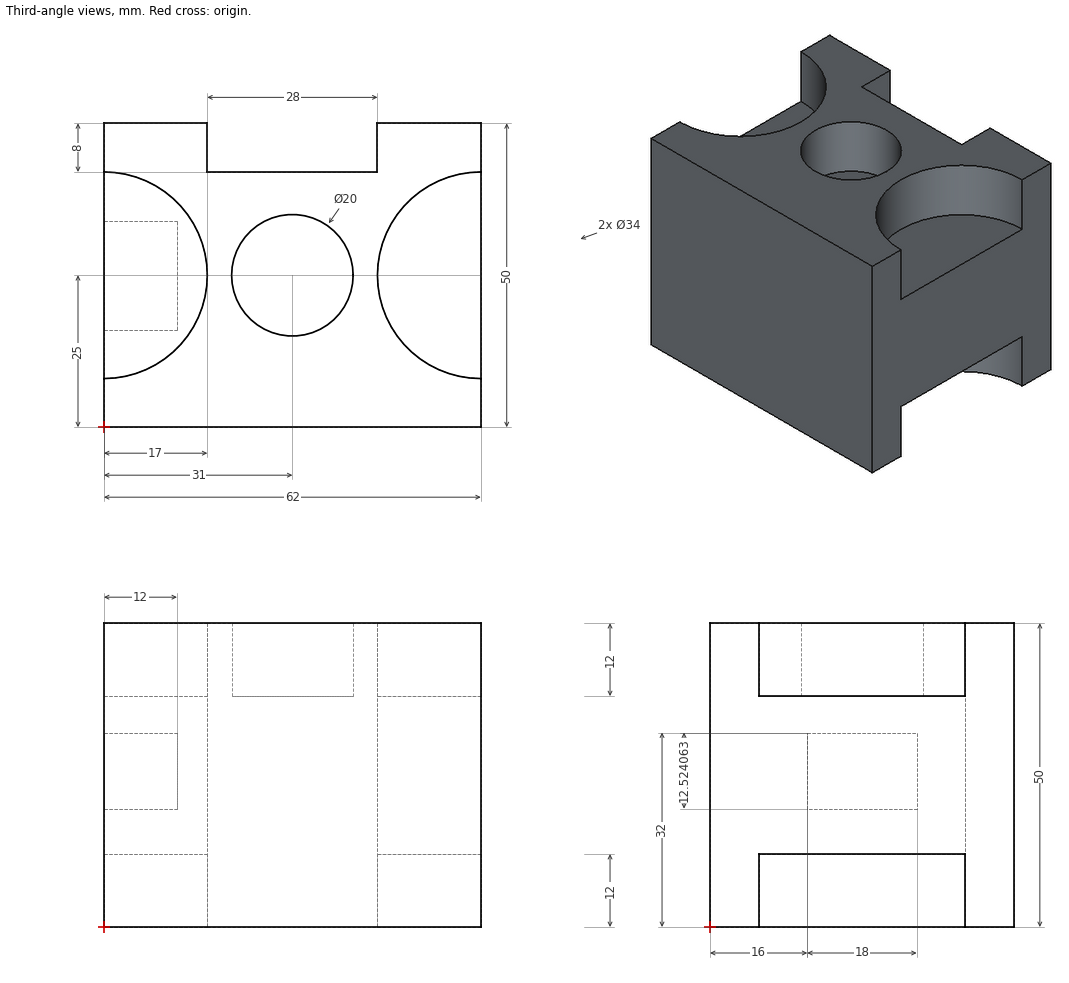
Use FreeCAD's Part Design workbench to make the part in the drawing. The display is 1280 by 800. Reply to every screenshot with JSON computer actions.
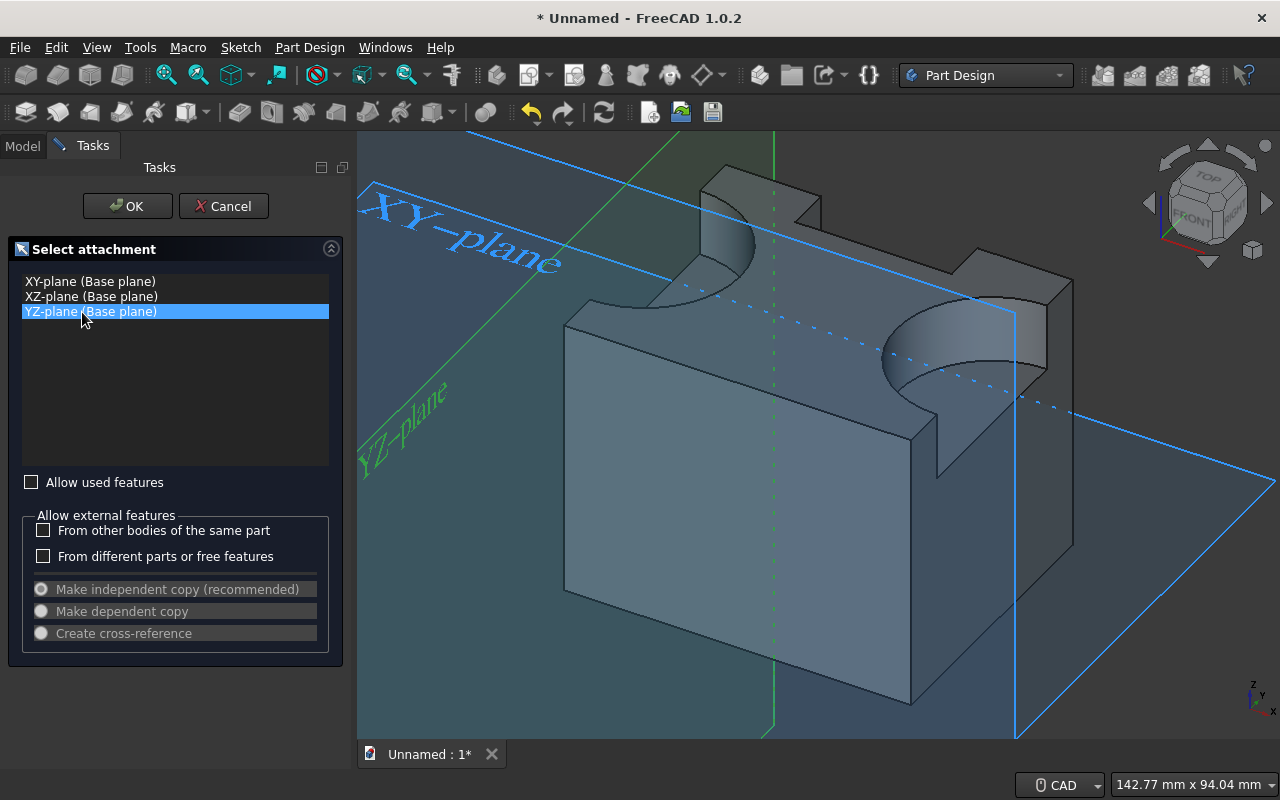
{"action": "left_click", "coordinate": [128, 206]}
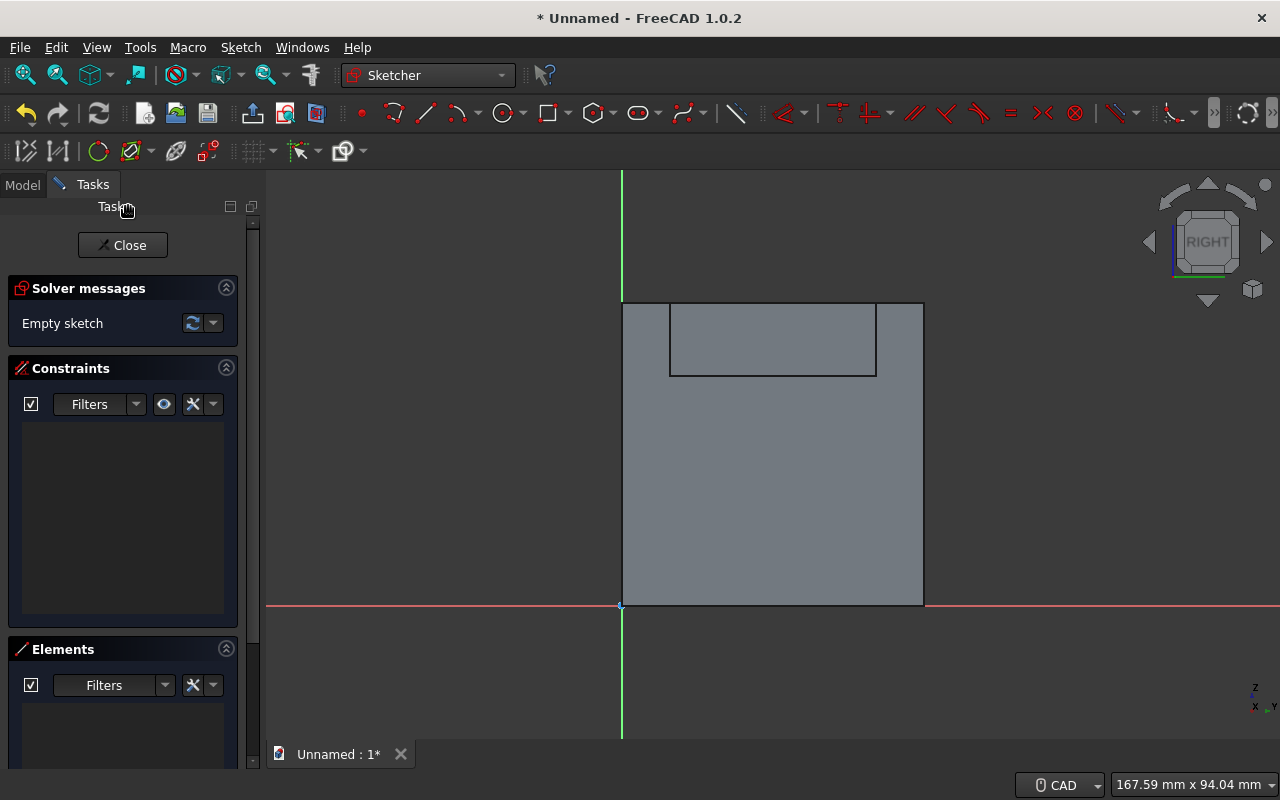
{"action": "left_click", "coordinate": [318, 114]}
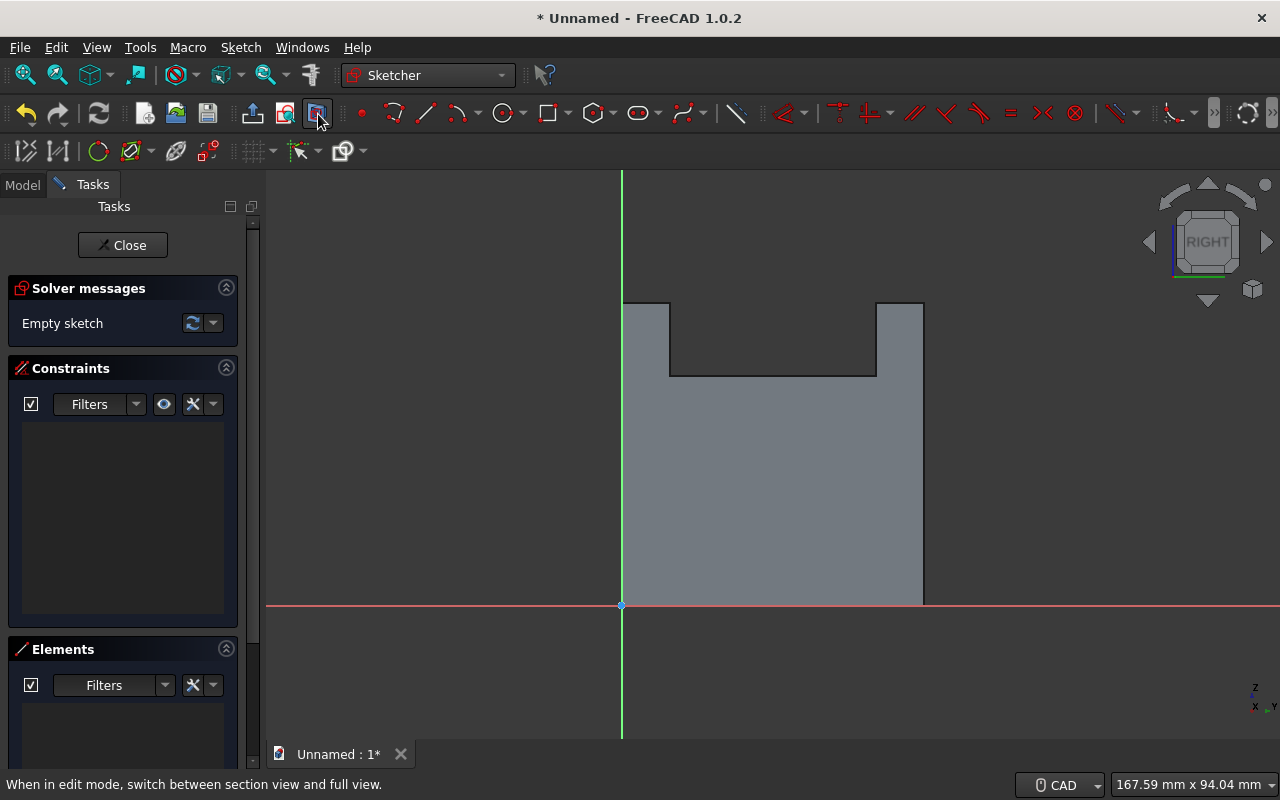
{"action": "scroll", "coordinate": [749, 575], "scroll_direction": "up", "scroll_amount": 3}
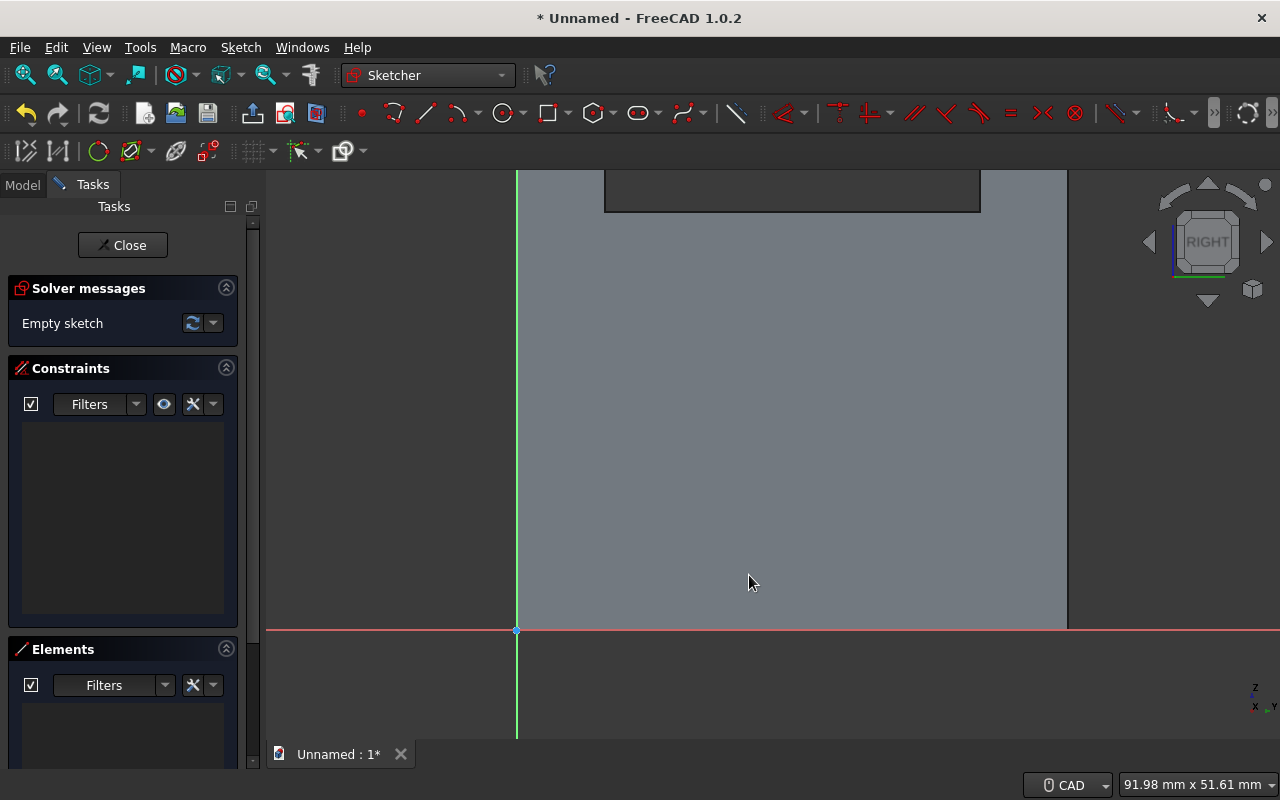
{"action": "left_click", "coordinate": [548, 114]}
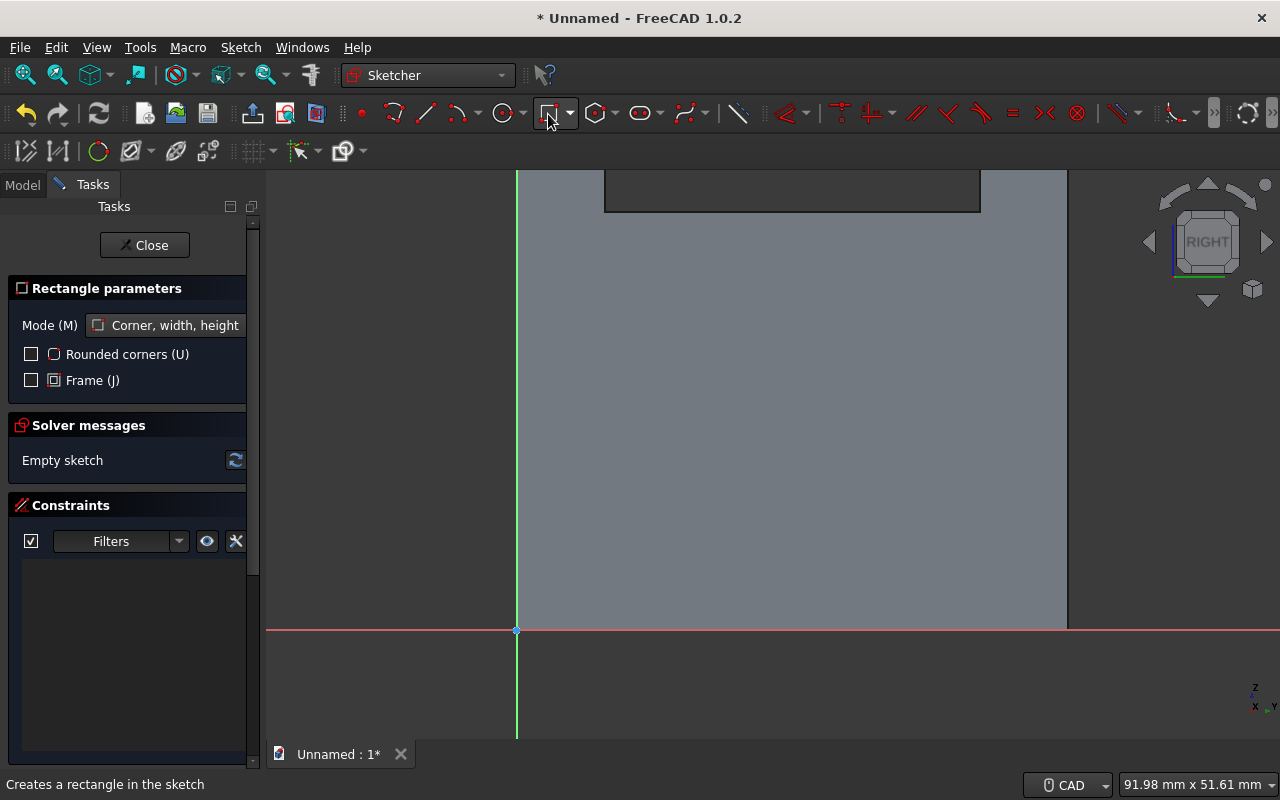
{"action": "left_click", "coordinate": [693, 278]}
{"action": "left_click", "coordinate": [892, 416]}
{"action": "key", "text": "Escape"}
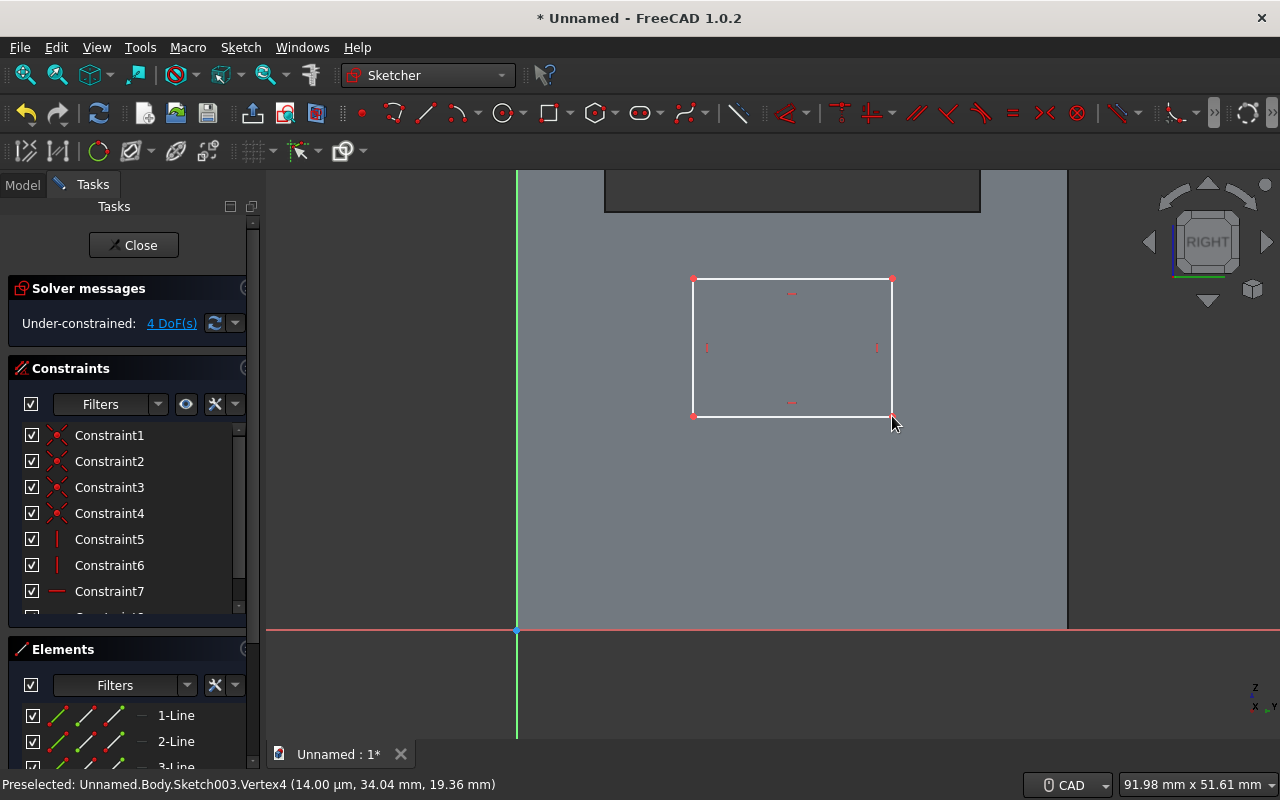
{"action": "left_click", "coordinate": [786, 114]}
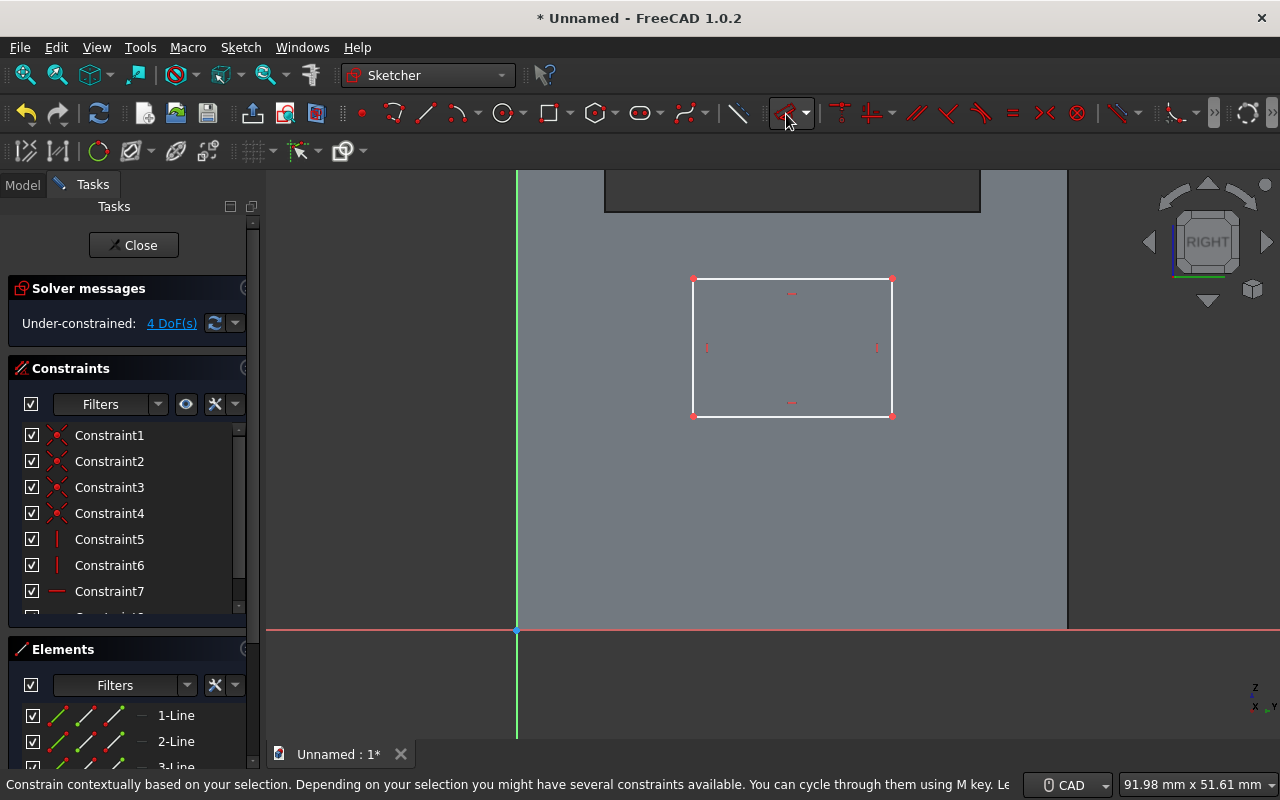
{"action": "left_click", "coordinate": [753, 417]}
{"action": "left_click", "coordinate": [793, 383]}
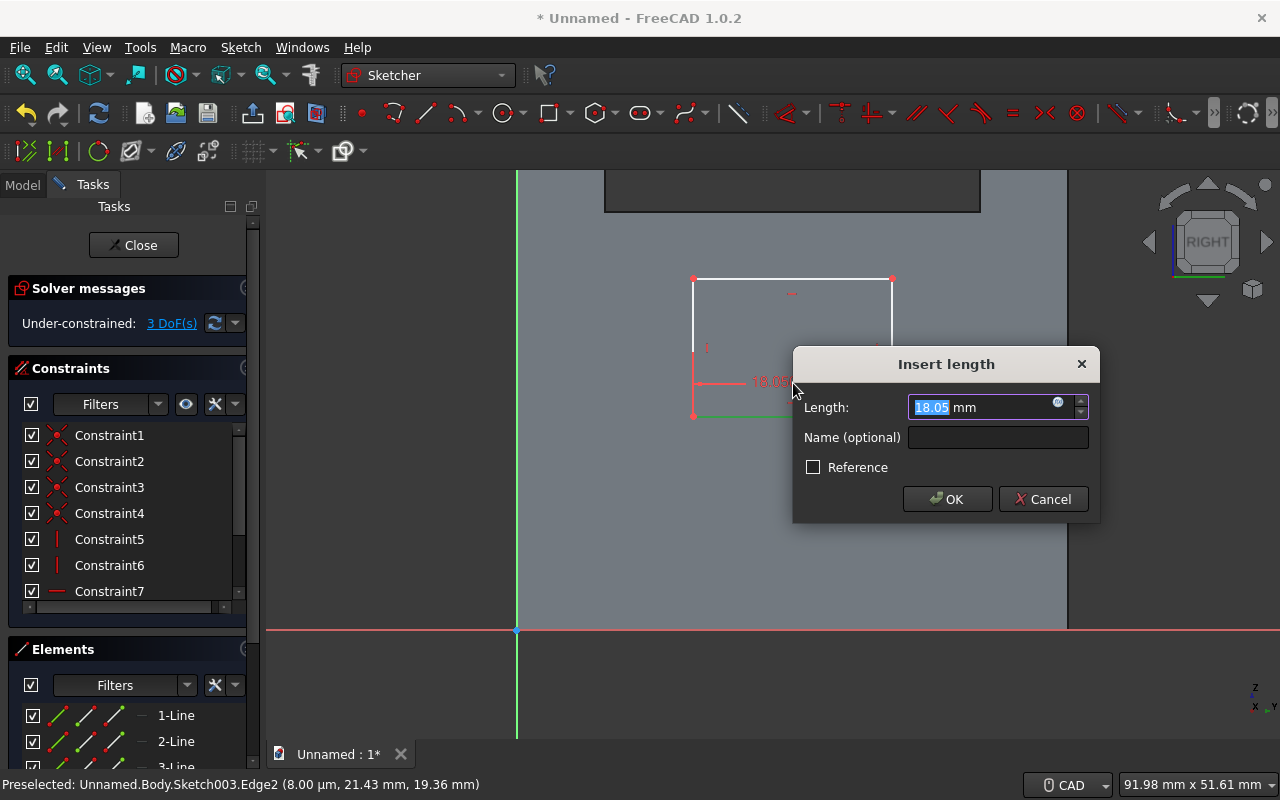
{"action": "type", "text": "18"}
{"action": "key", "text": "Return"}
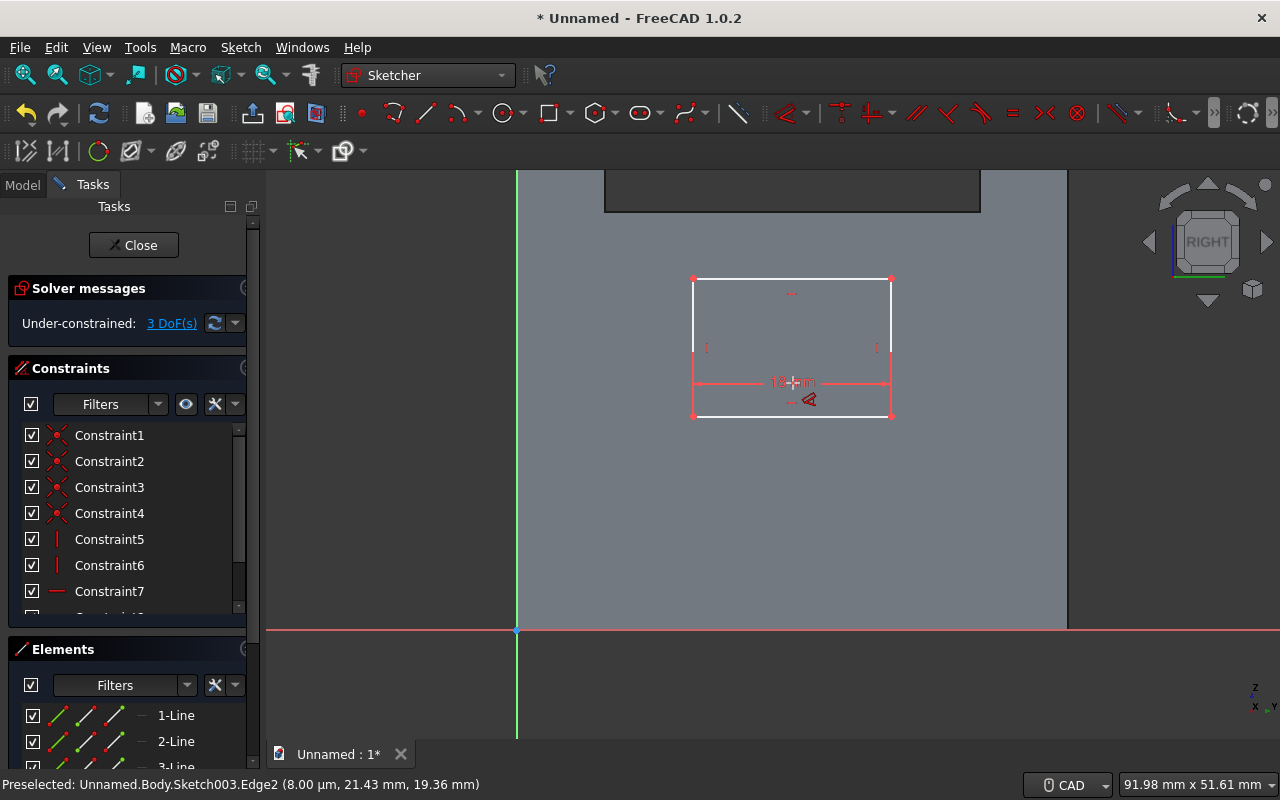
{"action": "left_click", "coordinate": [693, 279]}
{"action": "left_click", "coordinate": [605, 664]}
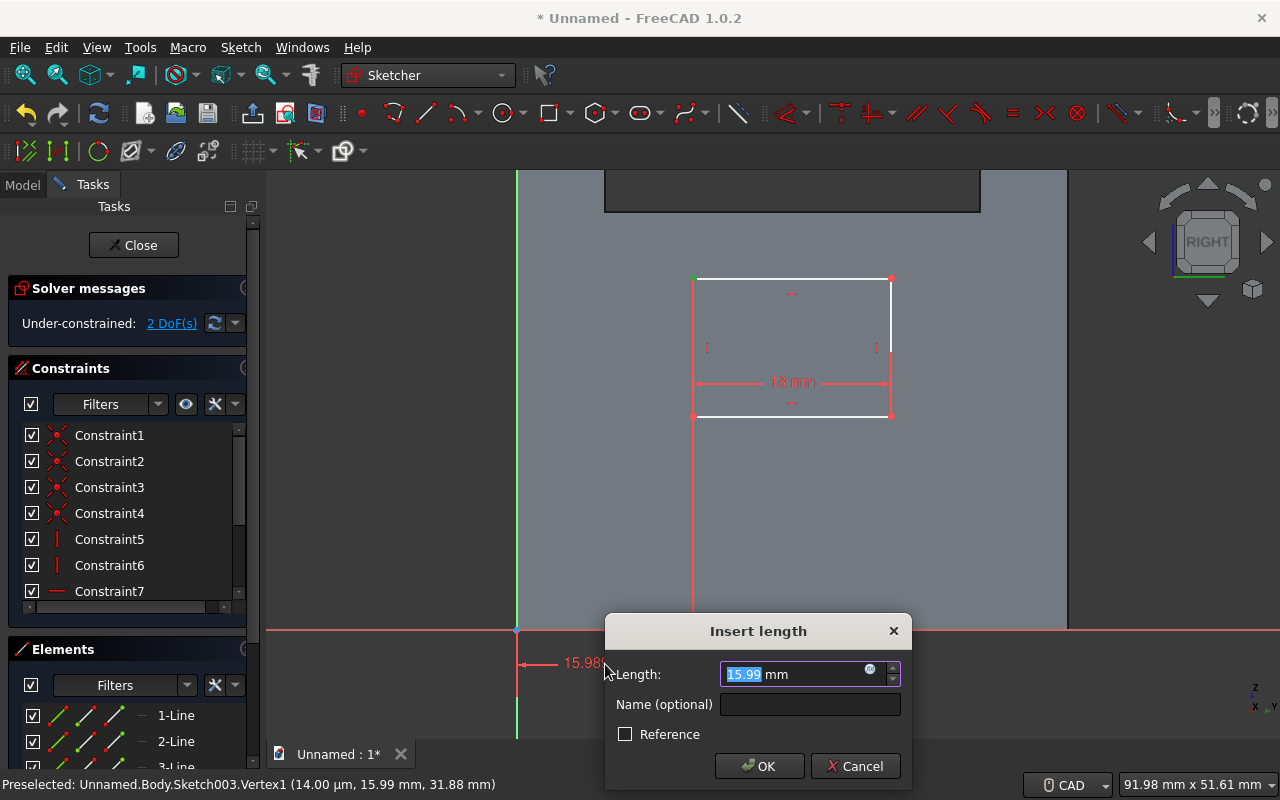
{"action": "type", "text": "16"}
{"action": "key", "text": "Return"}